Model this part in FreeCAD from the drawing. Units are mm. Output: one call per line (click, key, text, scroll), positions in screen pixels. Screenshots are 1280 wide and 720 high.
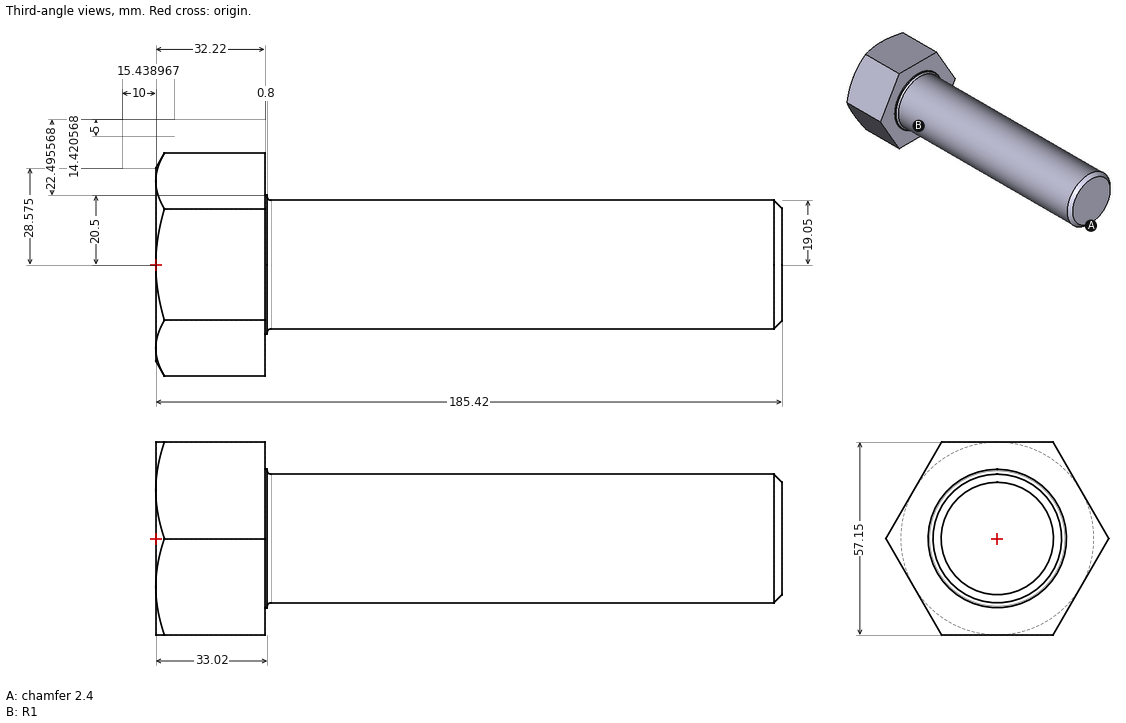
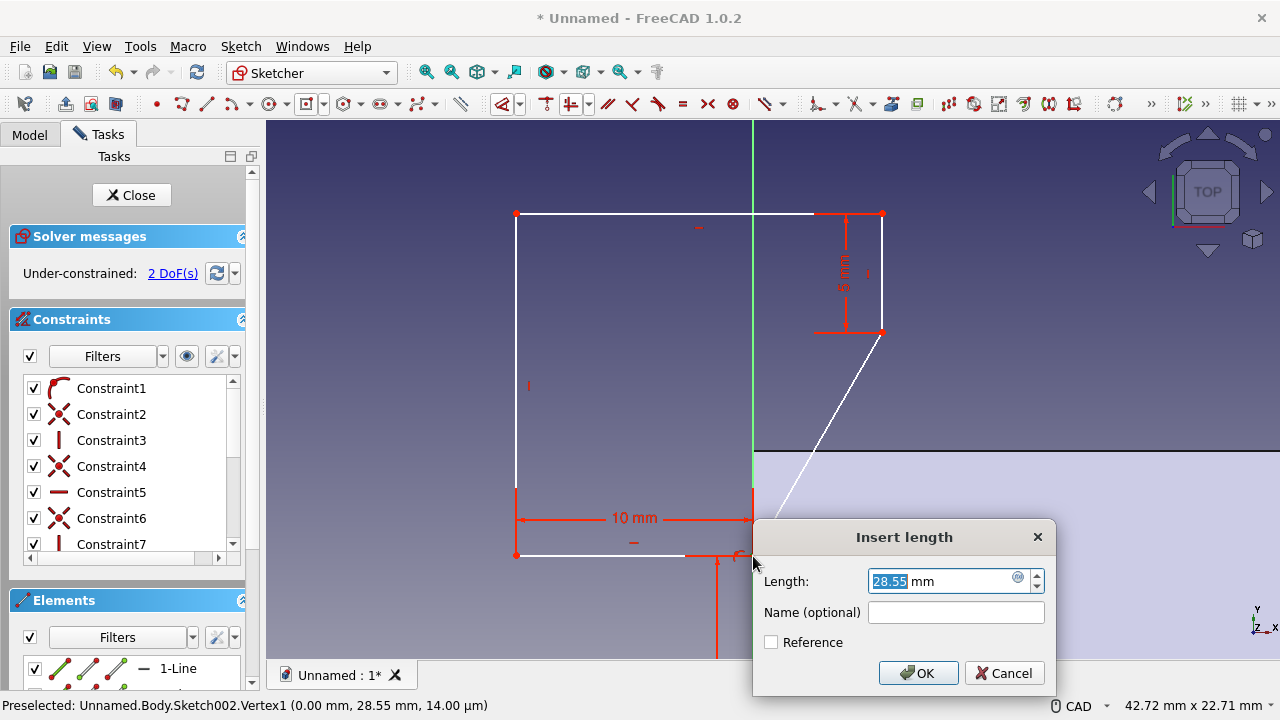
text(28.575)
key(Return)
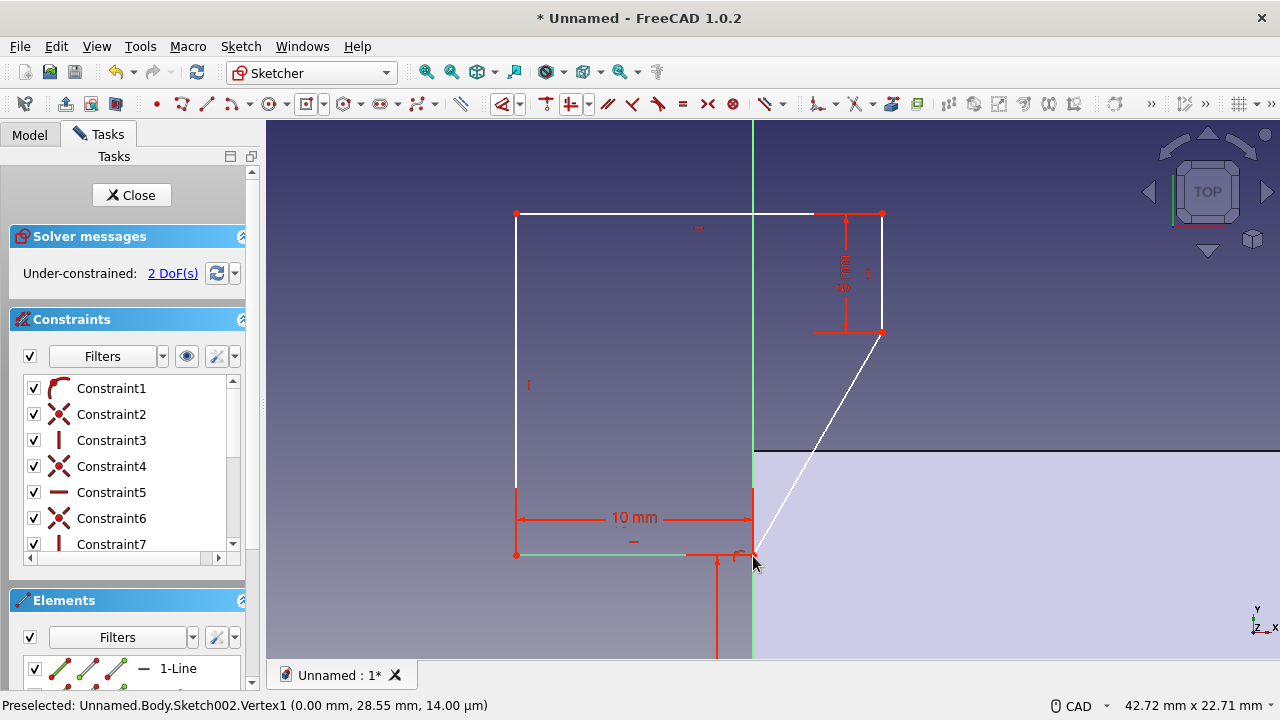
click(772, 214)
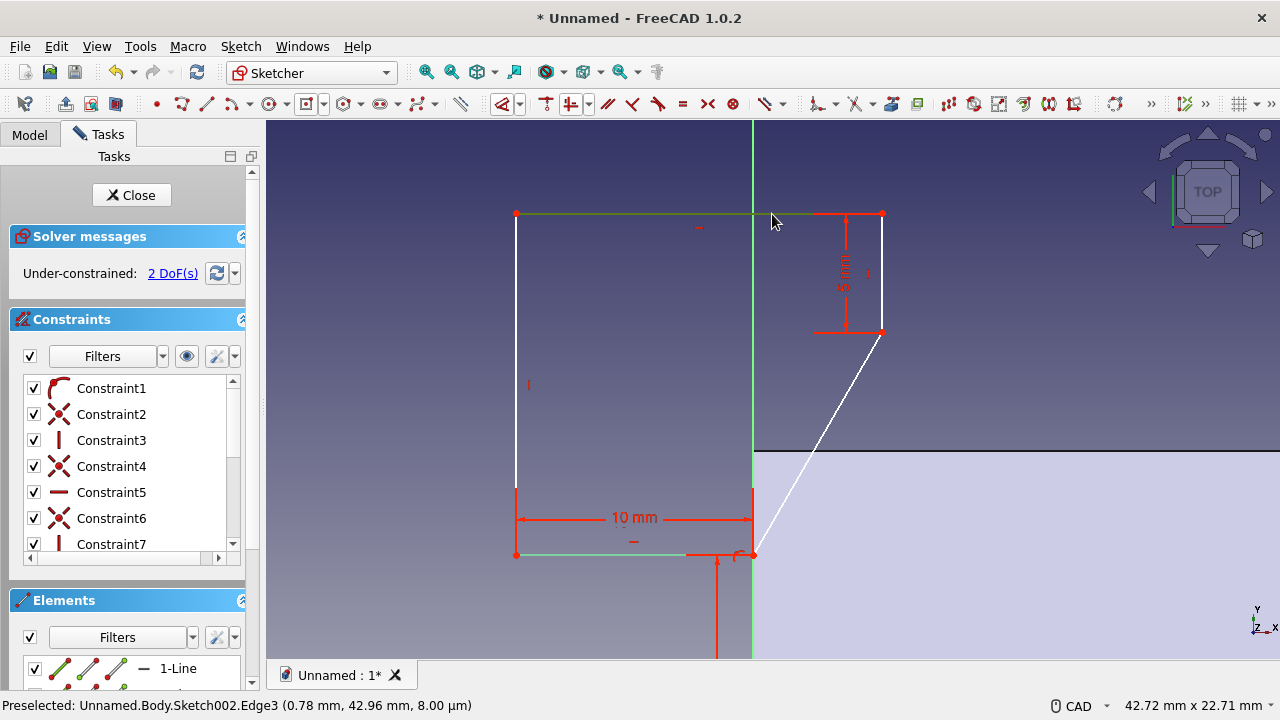
click(520, 104)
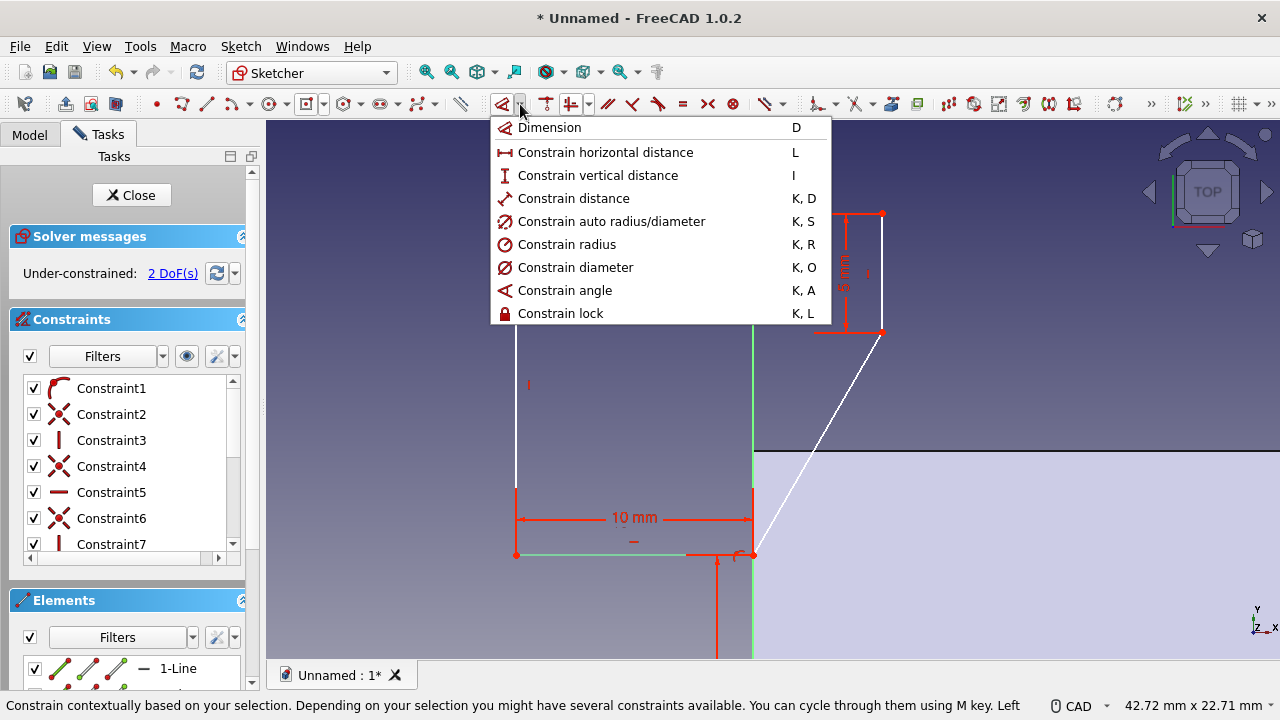
click(661, 152)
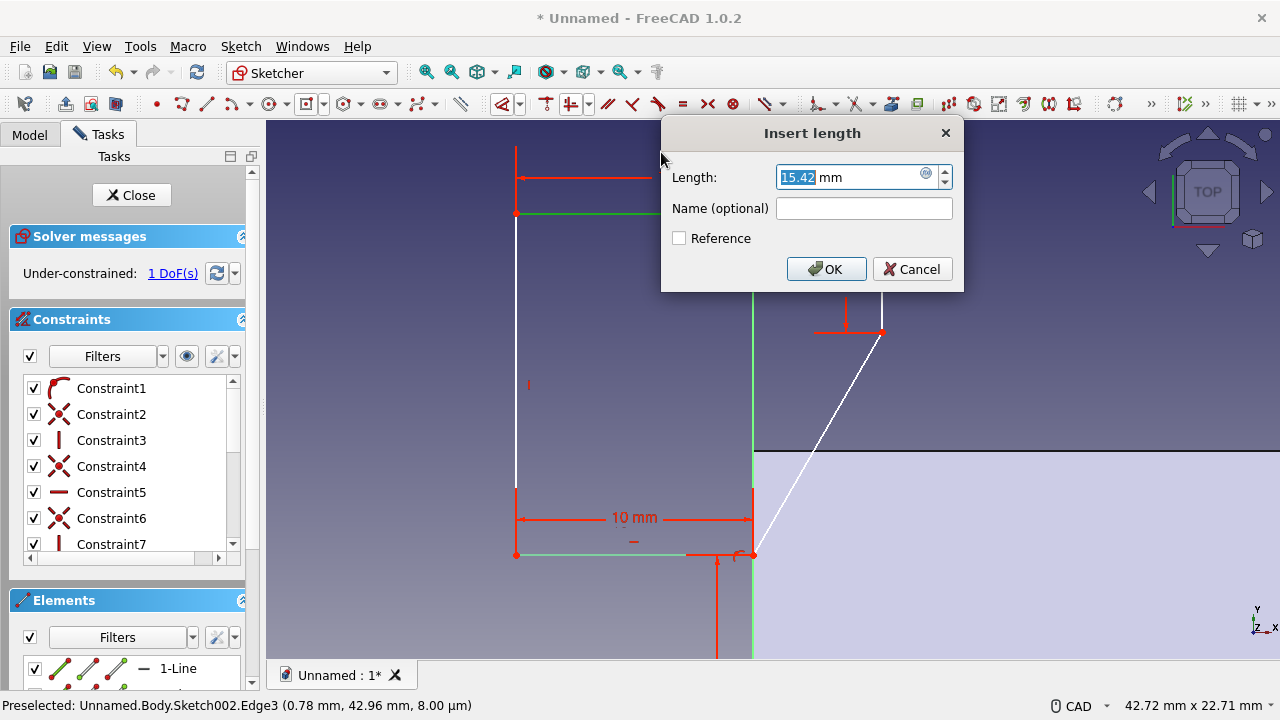
text(15.438967)
key(Return)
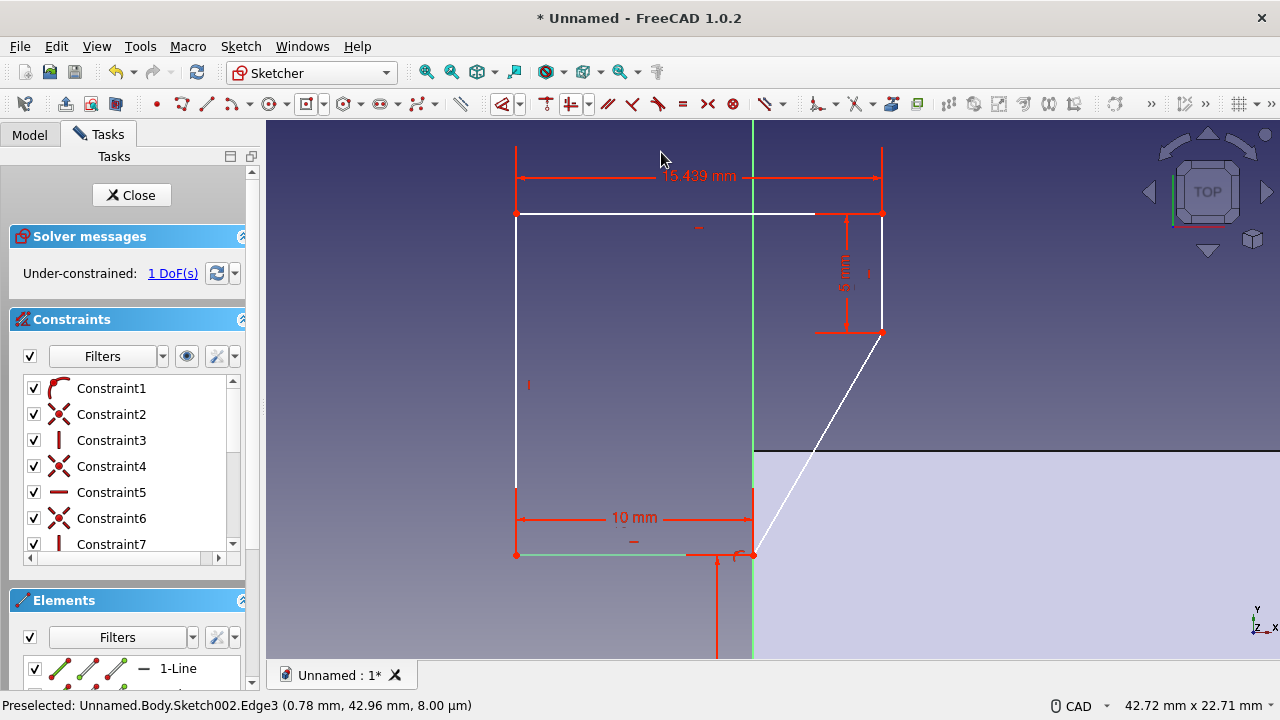
click(516, 316)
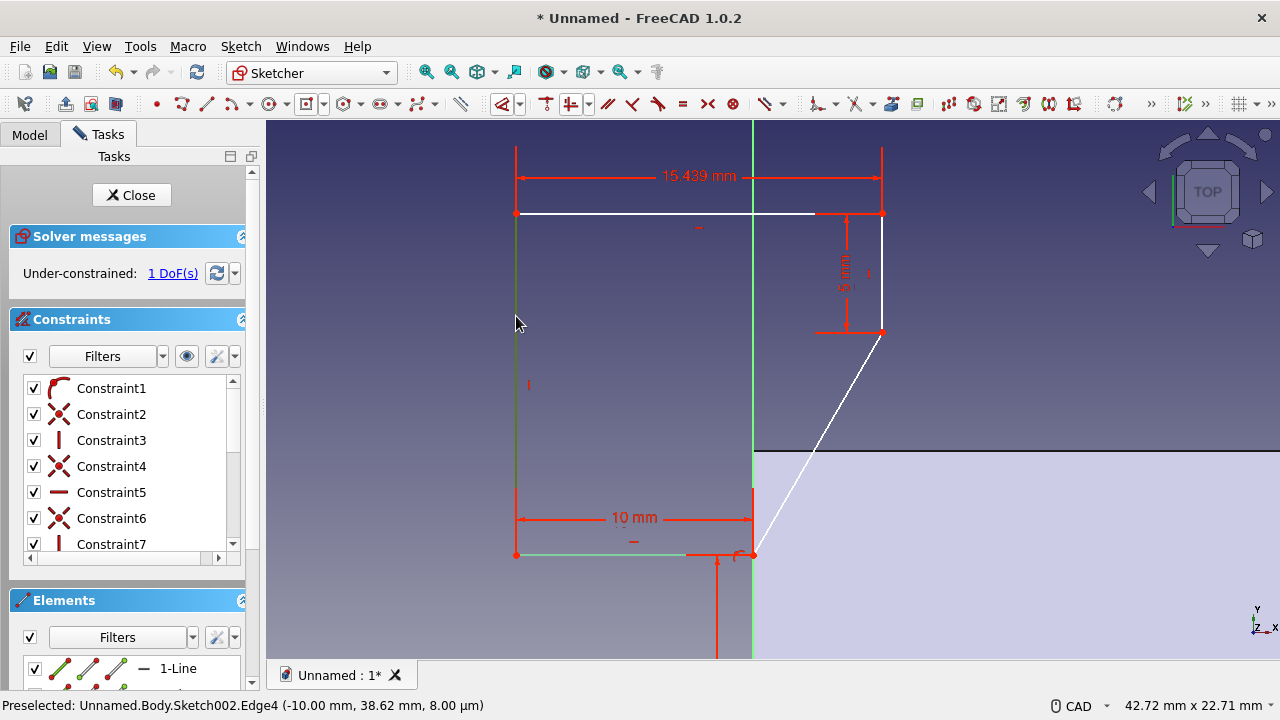
key(i)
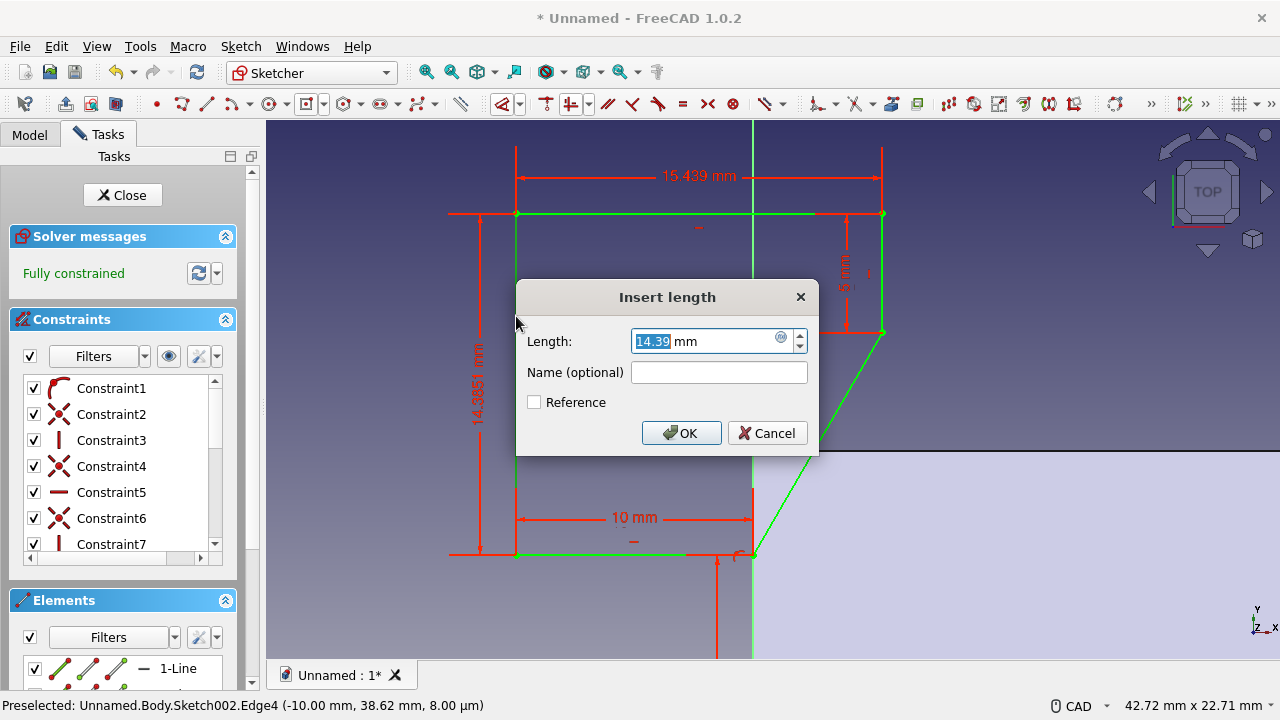
text(14.420568)
key(Return)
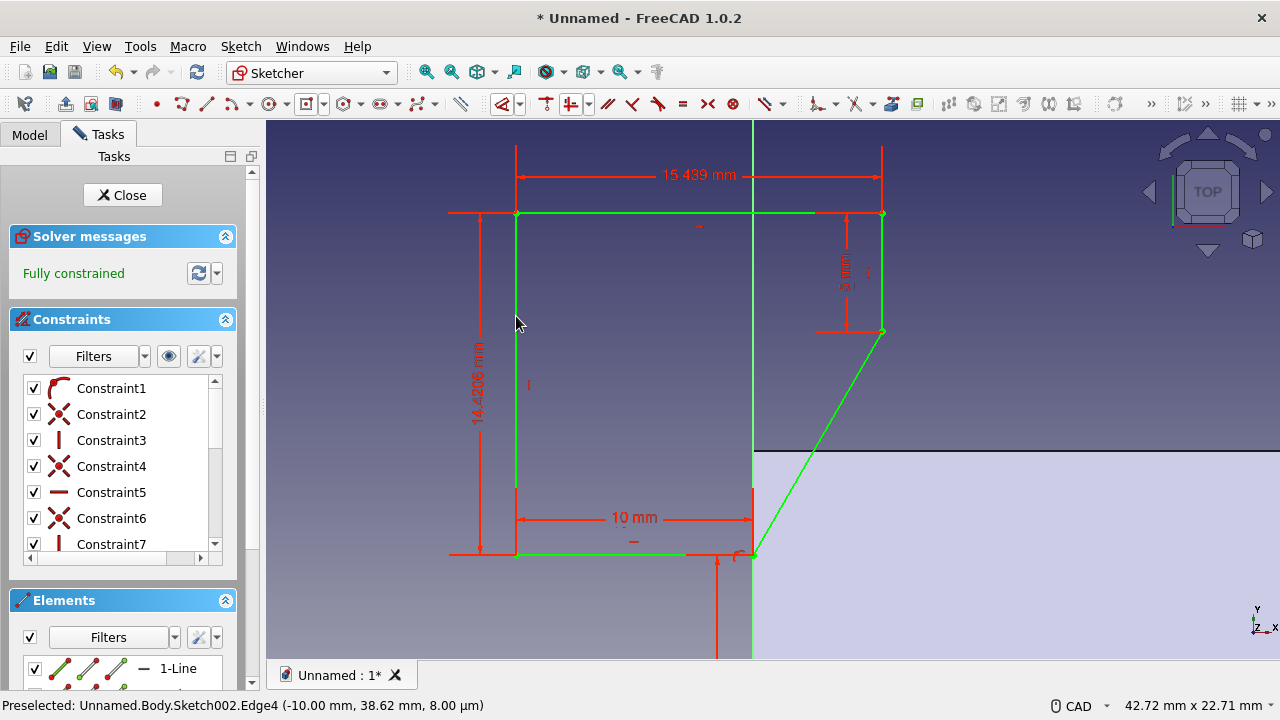
click(123, 195)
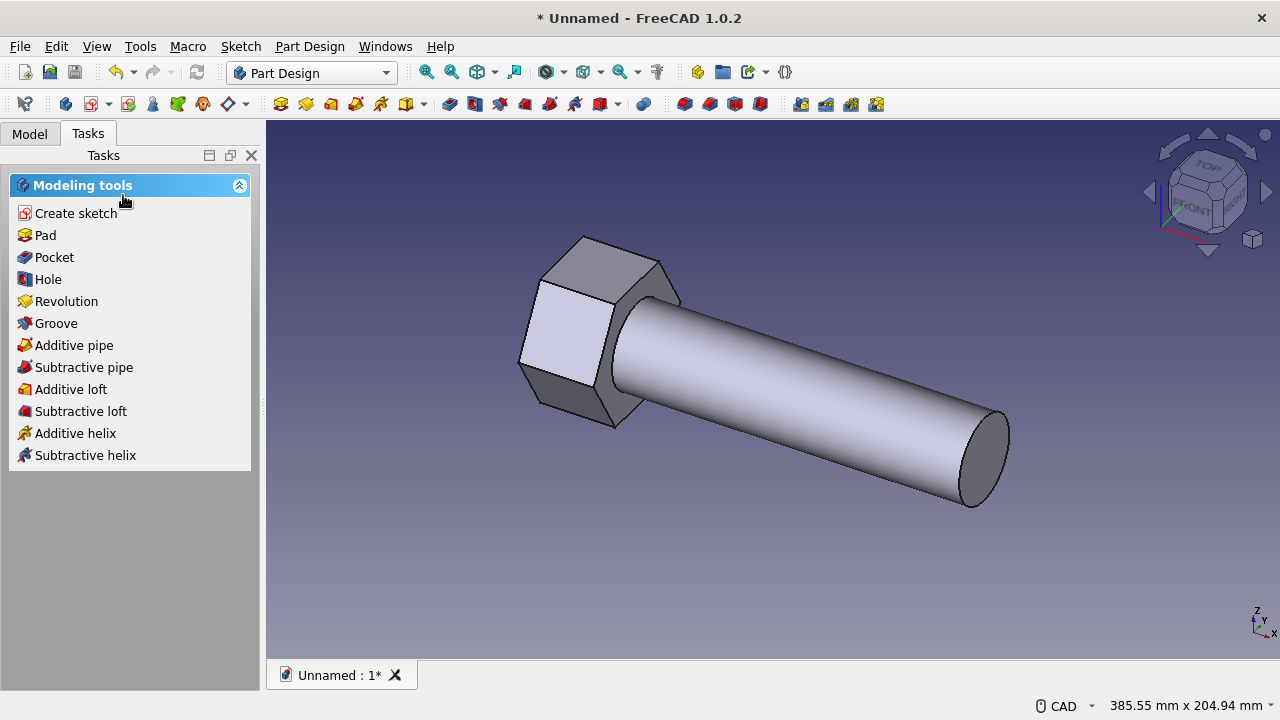
click(500, 104)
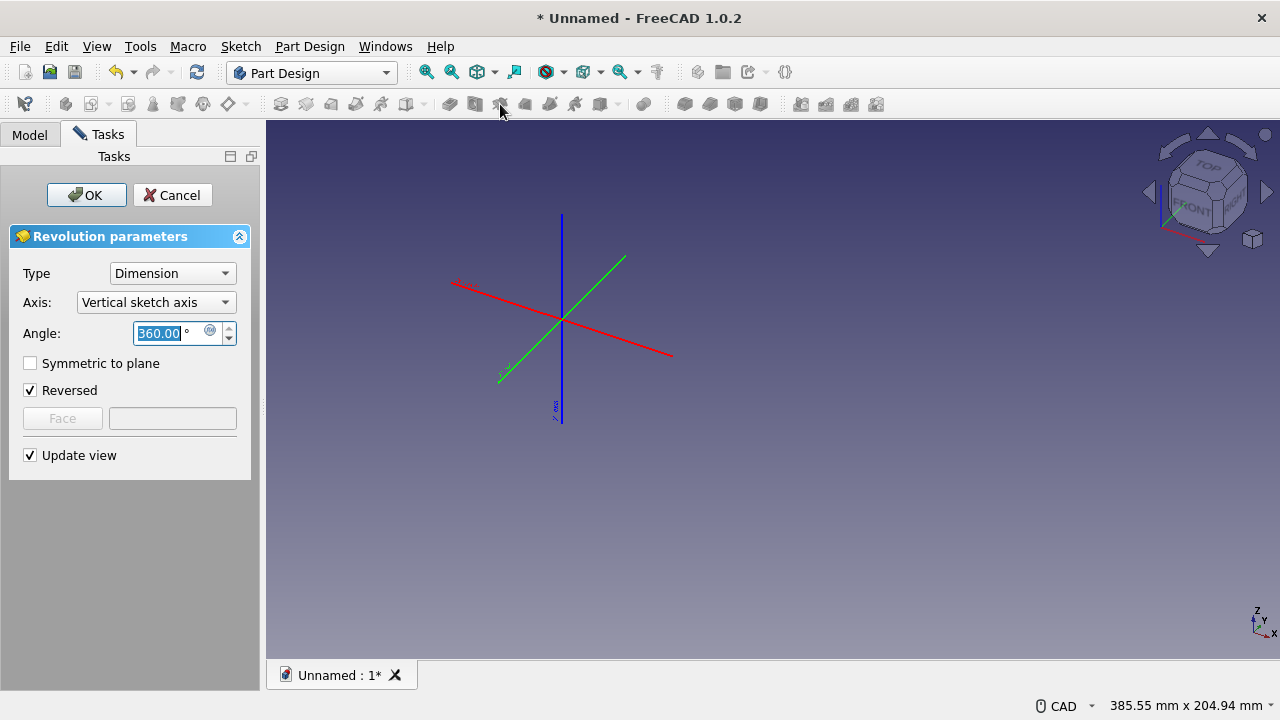
click(157, 302)